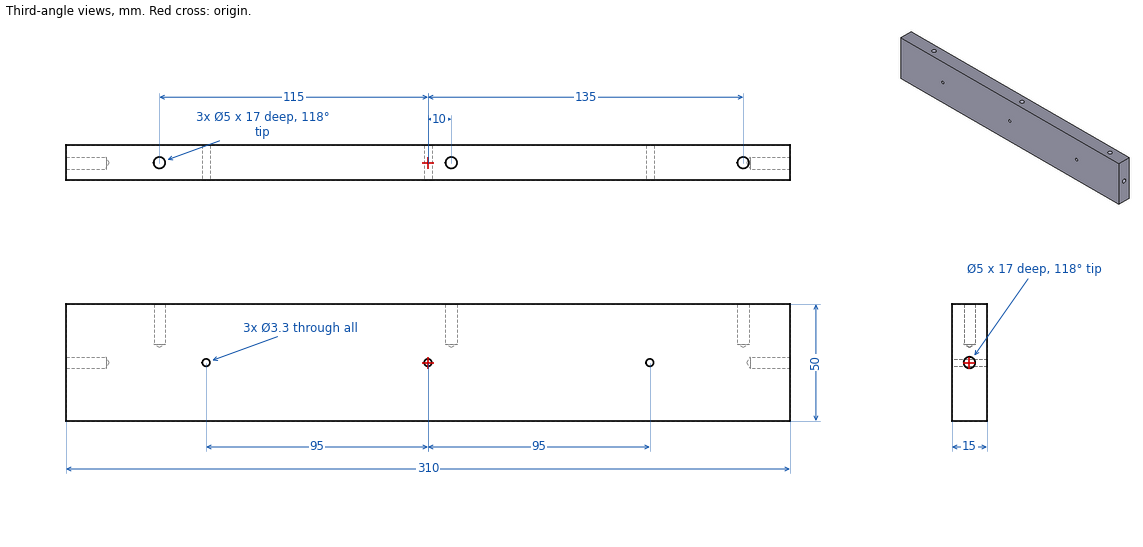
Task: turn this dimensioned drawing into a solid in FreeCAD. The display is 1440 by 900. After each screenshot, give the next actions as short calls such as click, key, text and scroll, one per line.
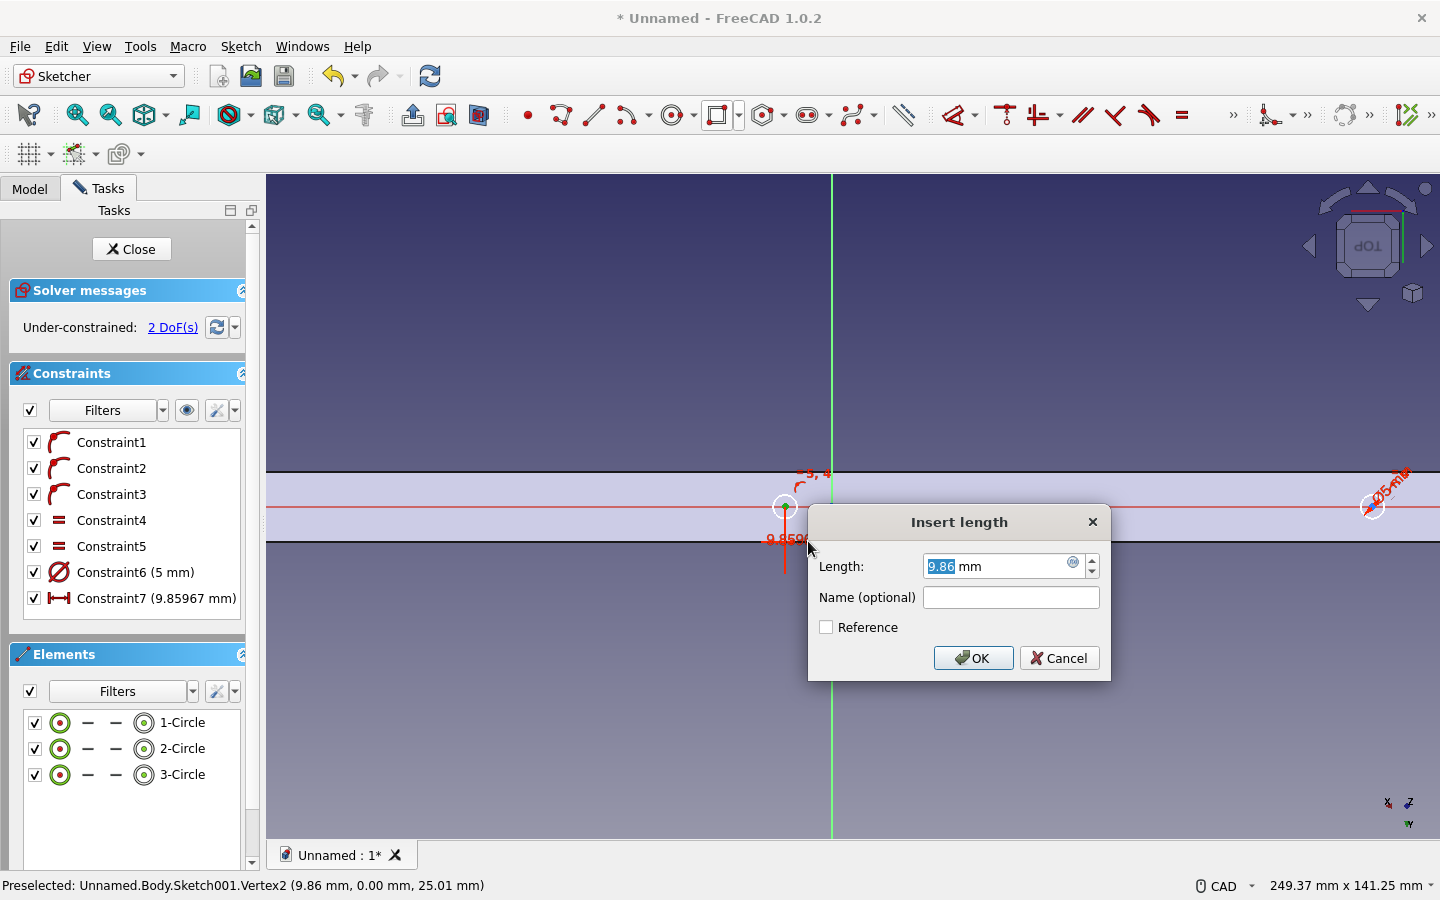
text(10)
key(Return)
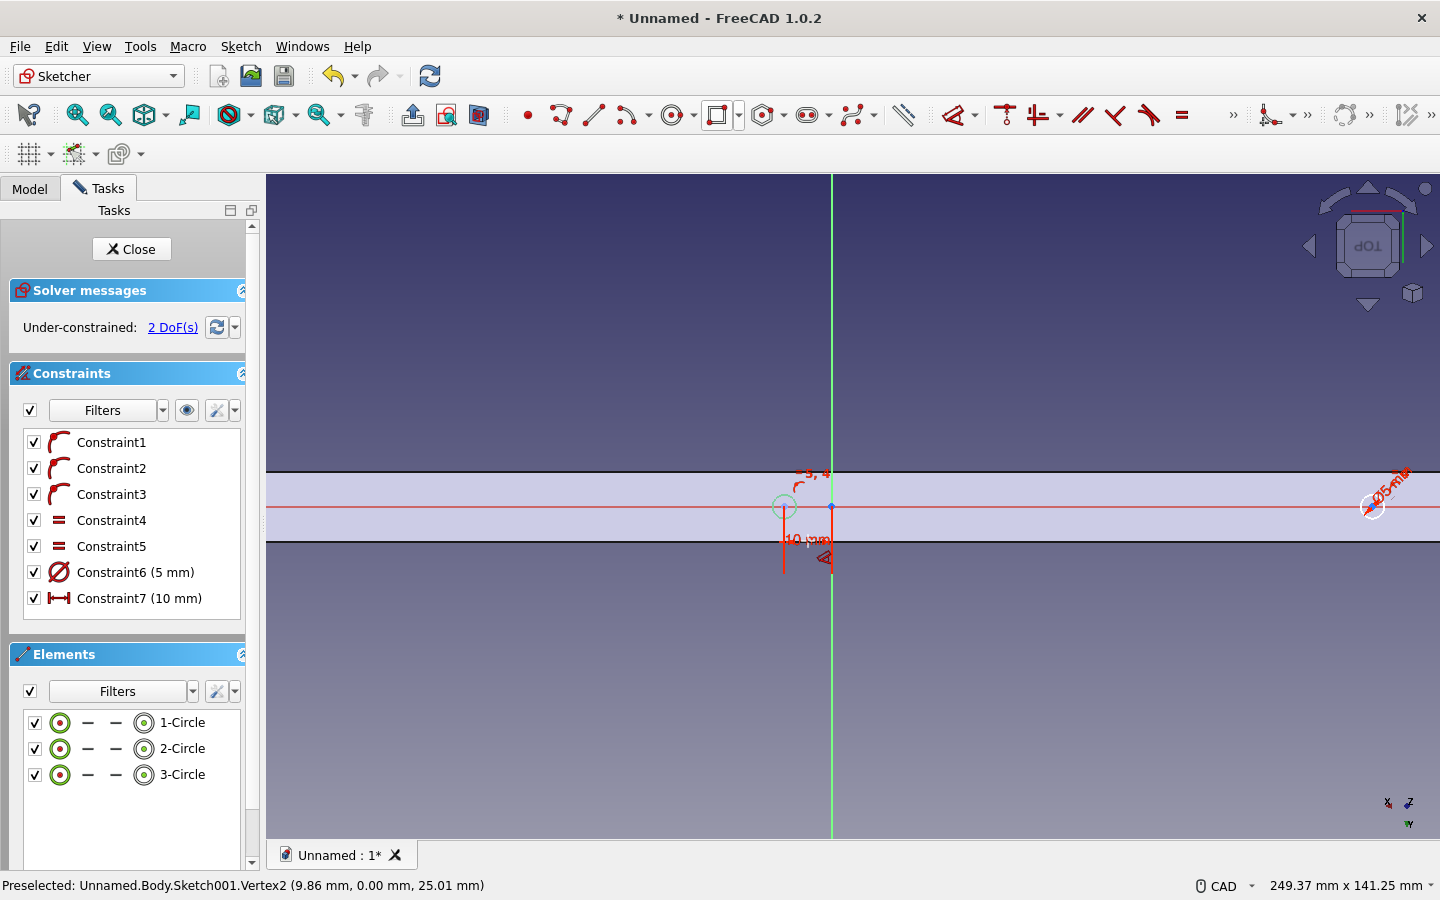
scroll(785, 506, down, 3)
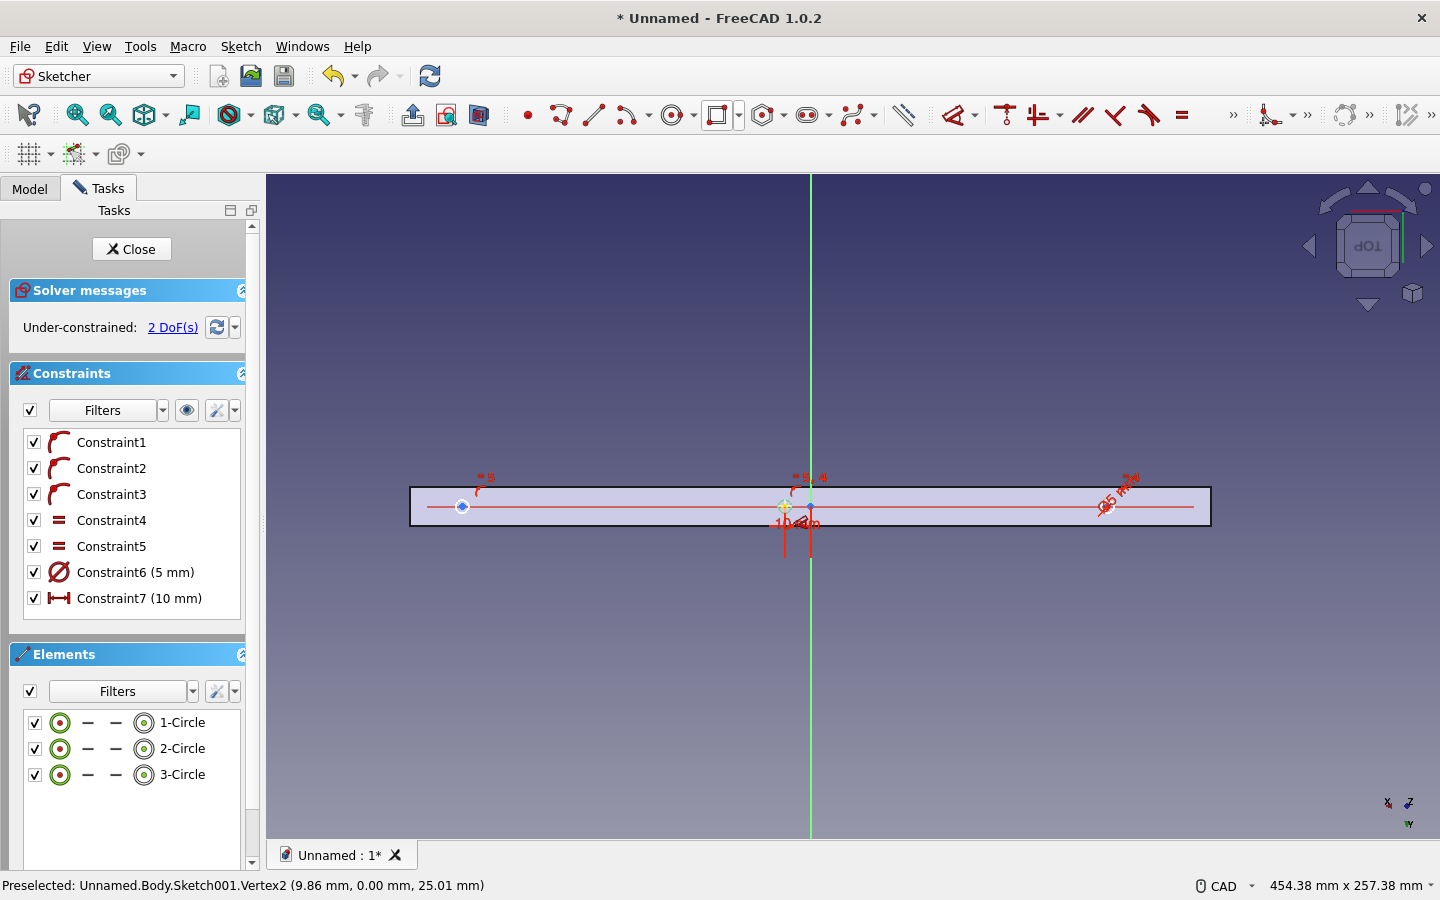
click(1108, 507)
click(959, 541)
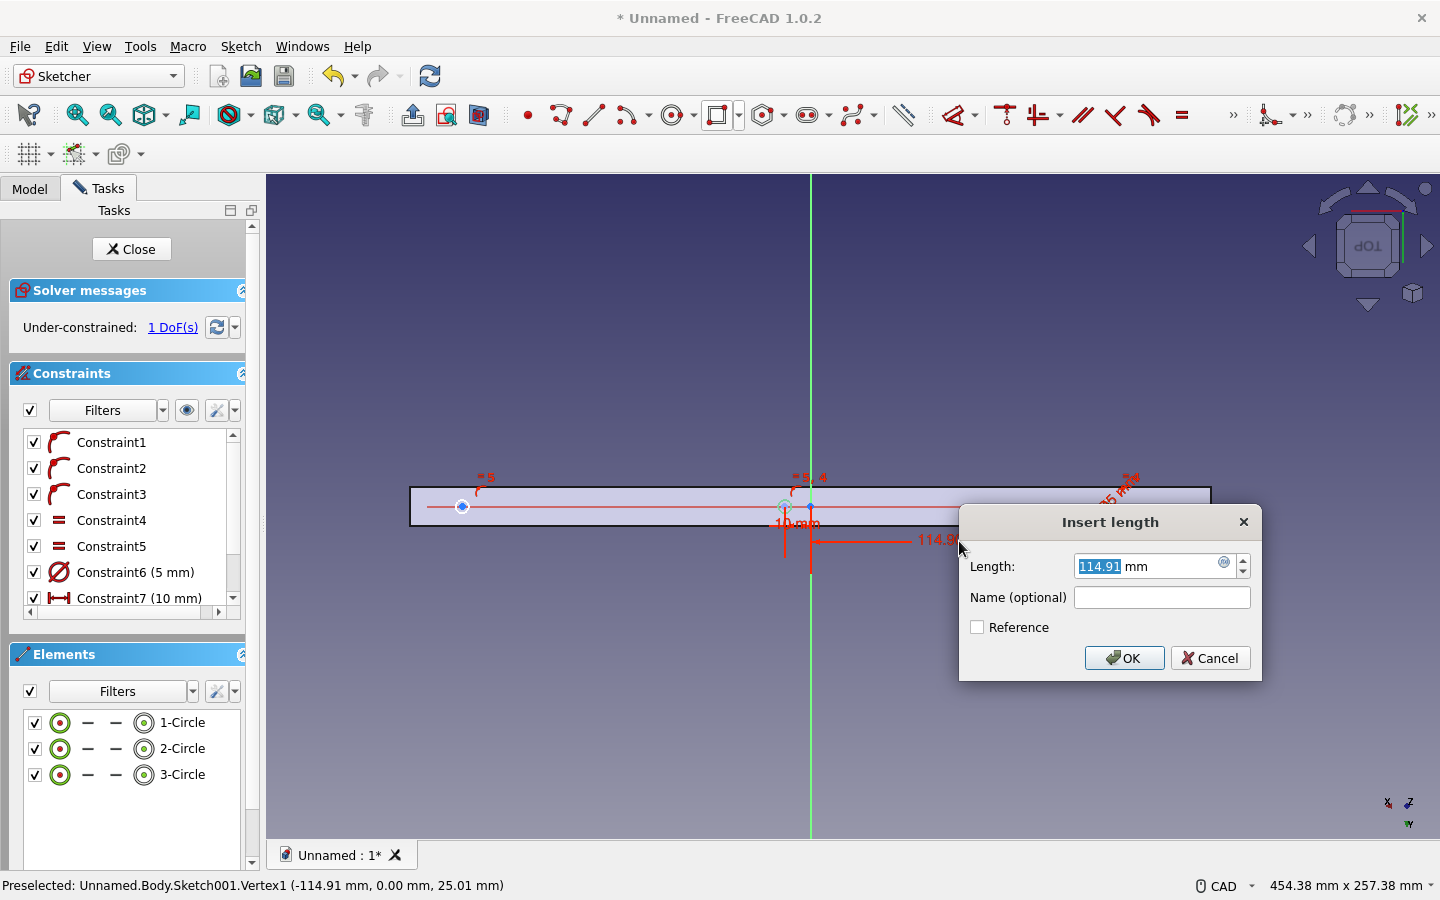
text(115)
key(Return)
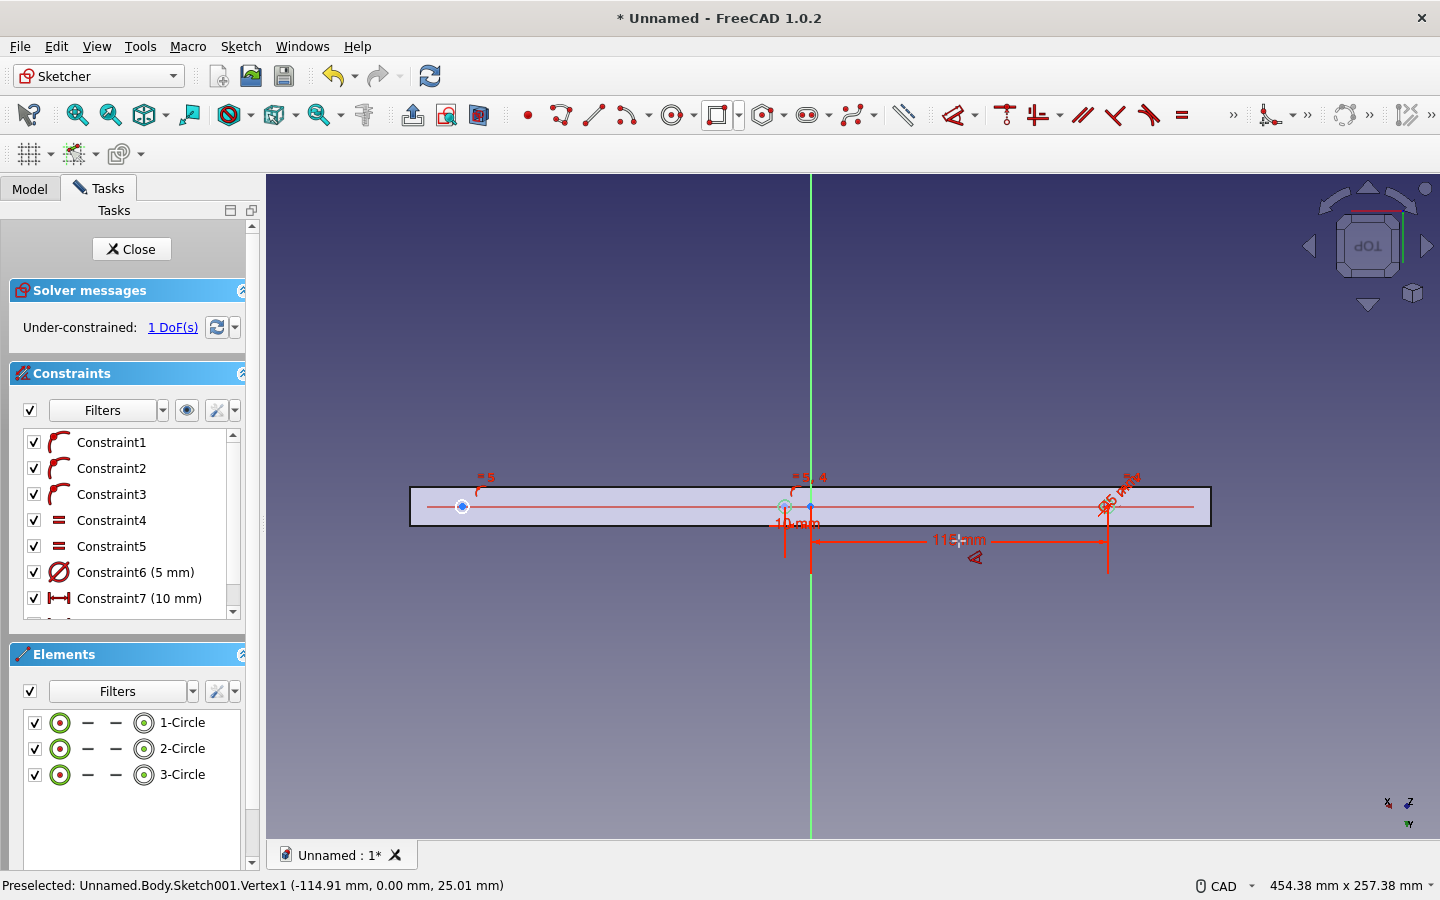
click(462, 507)
click(636, 541)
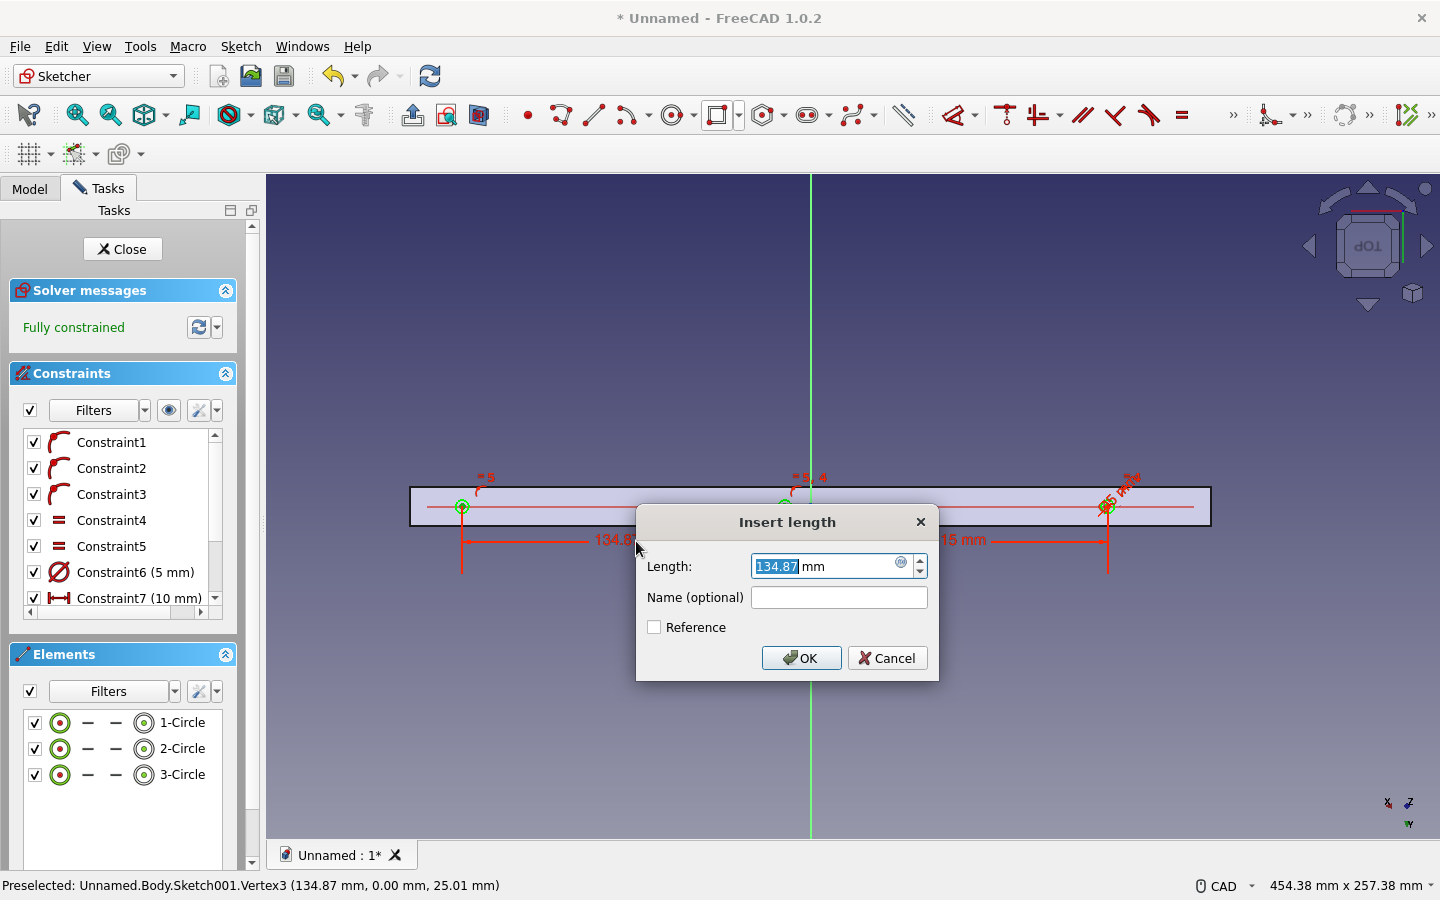
text(135)
key(Return)
key(Escape)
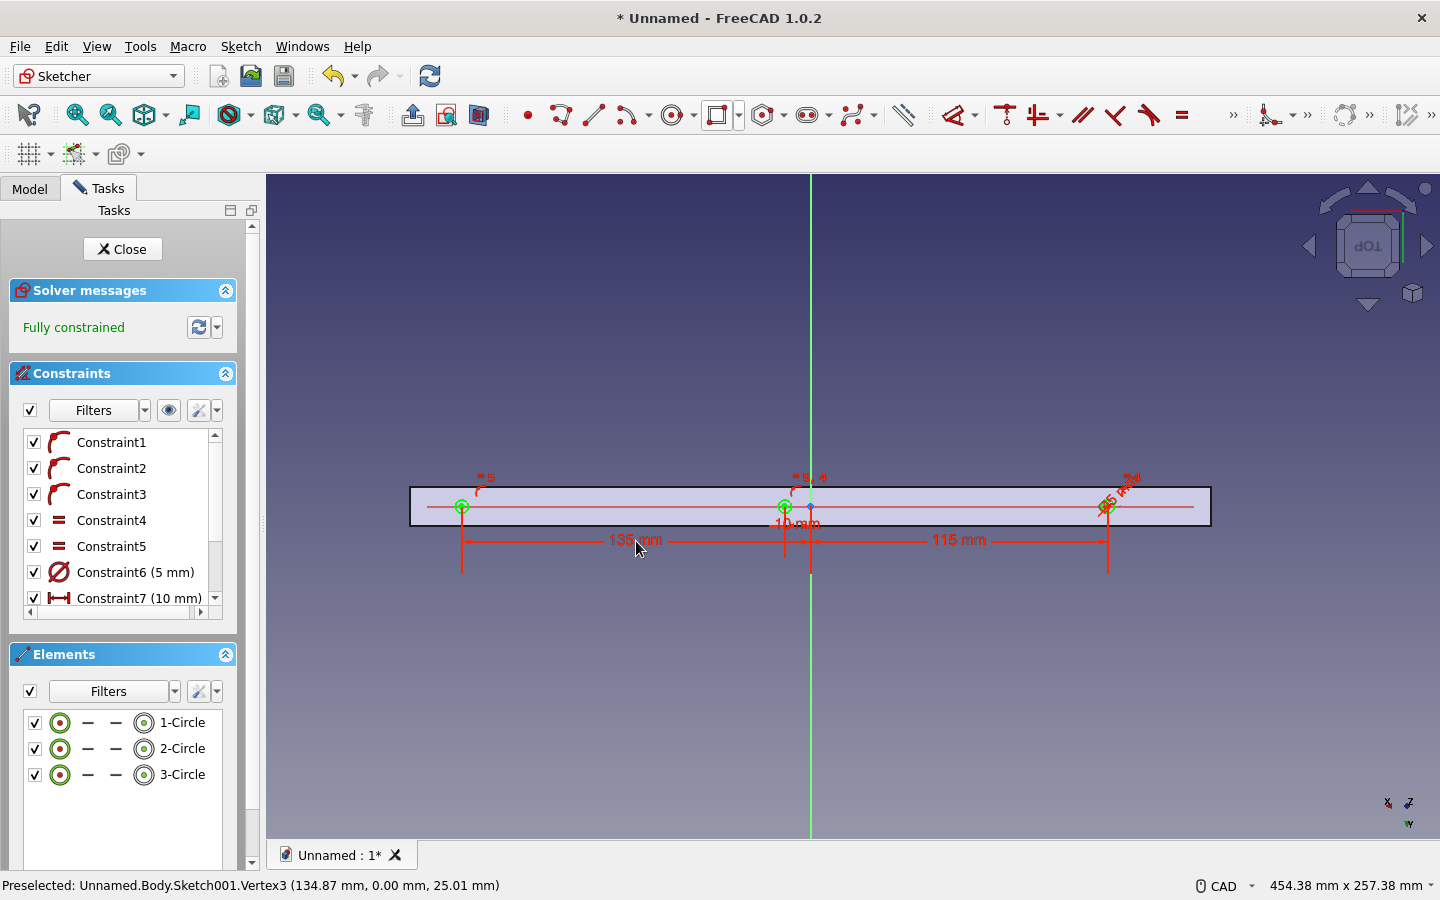
click(123, 249)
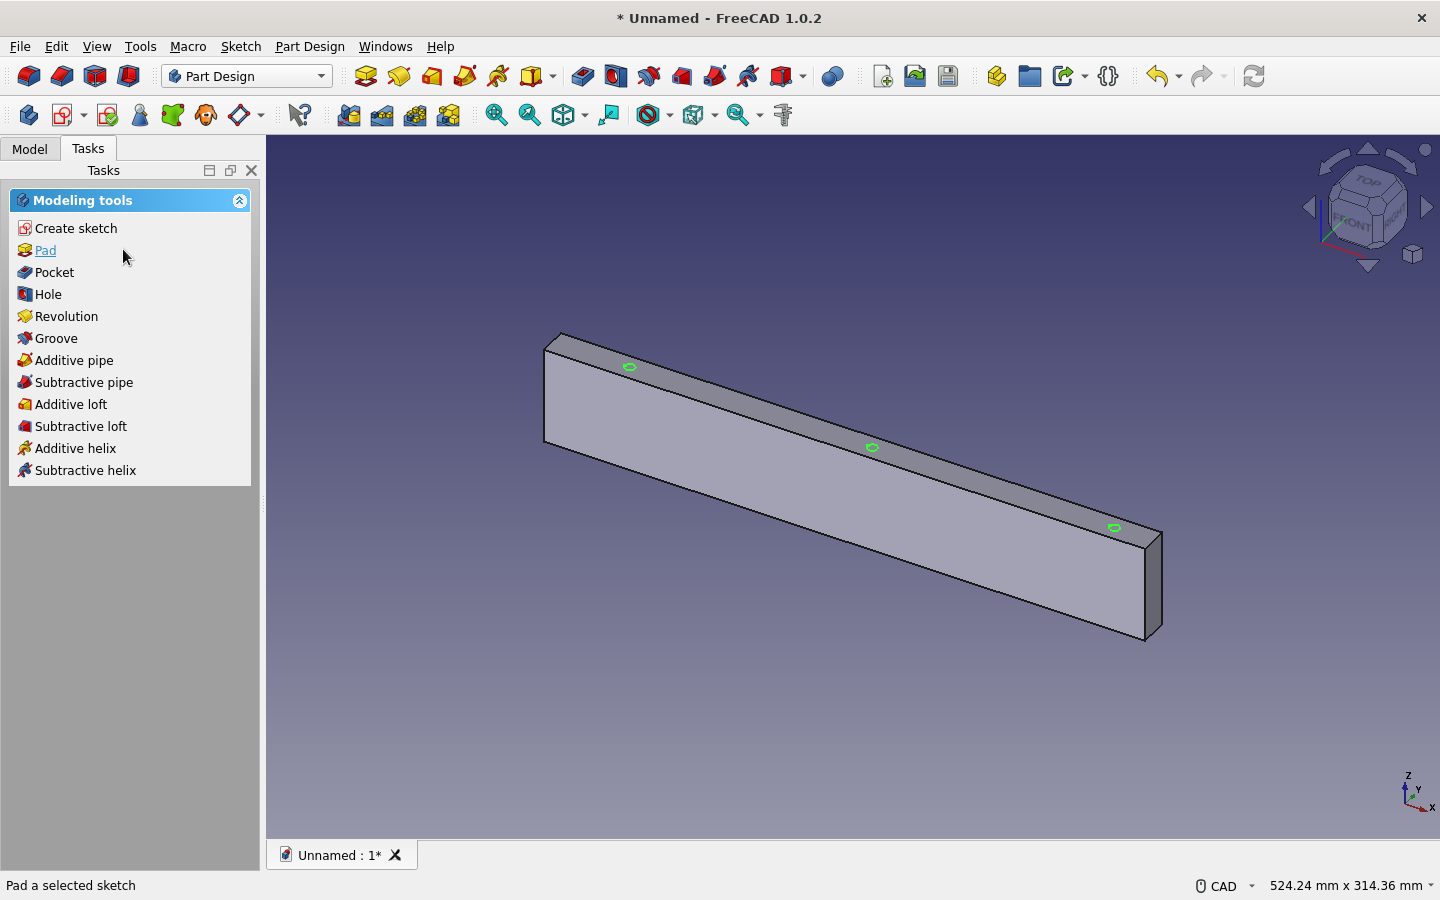
click(616, 76)